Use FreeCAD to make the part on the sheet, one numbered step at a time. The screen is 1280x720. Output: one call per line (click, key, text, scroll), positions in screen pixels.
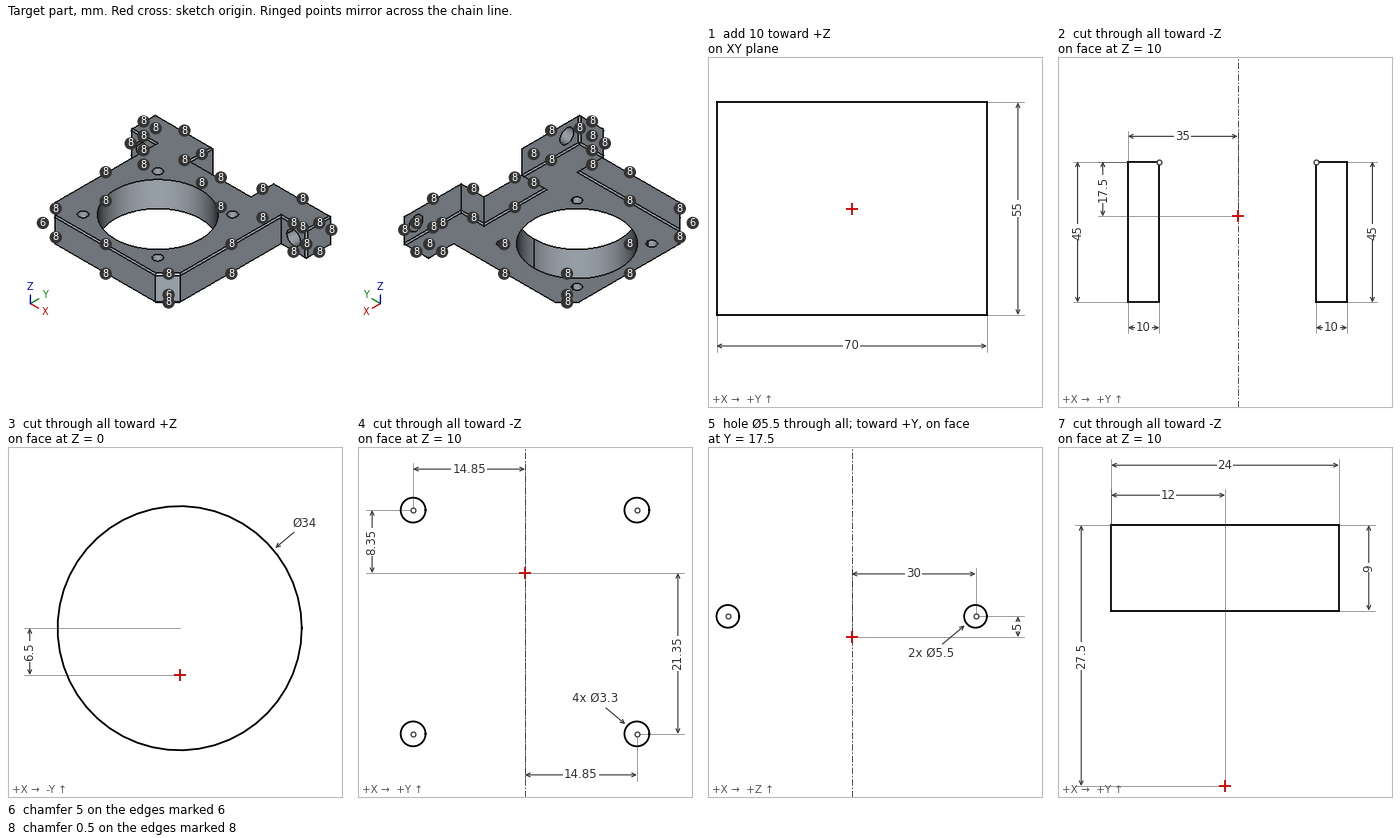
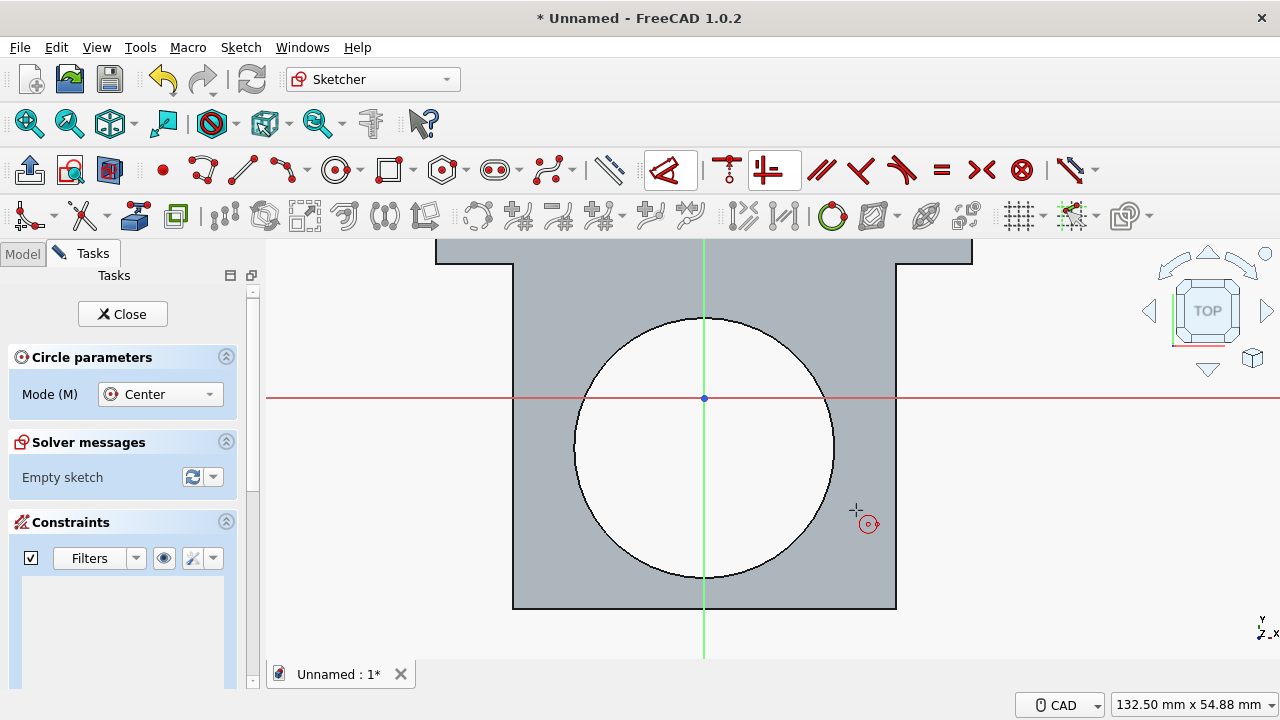
scroll(818, 562, up, 3)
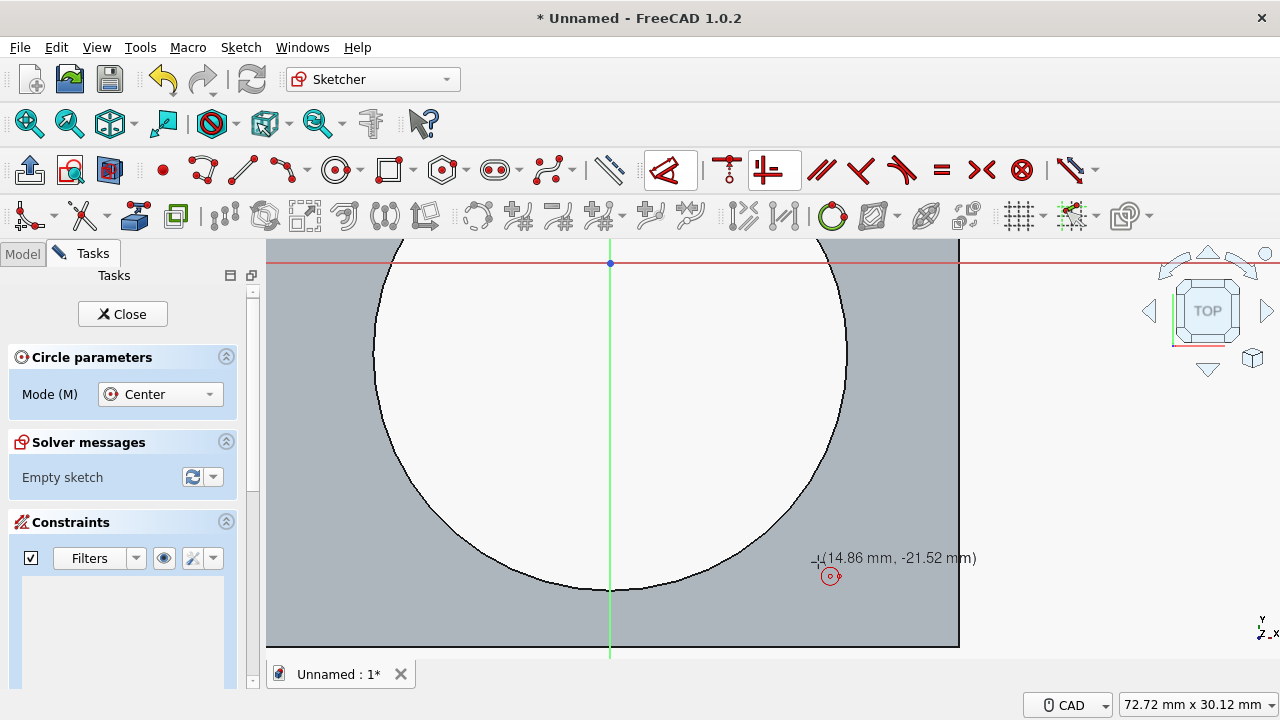
click(817, 561)
move(834, 545)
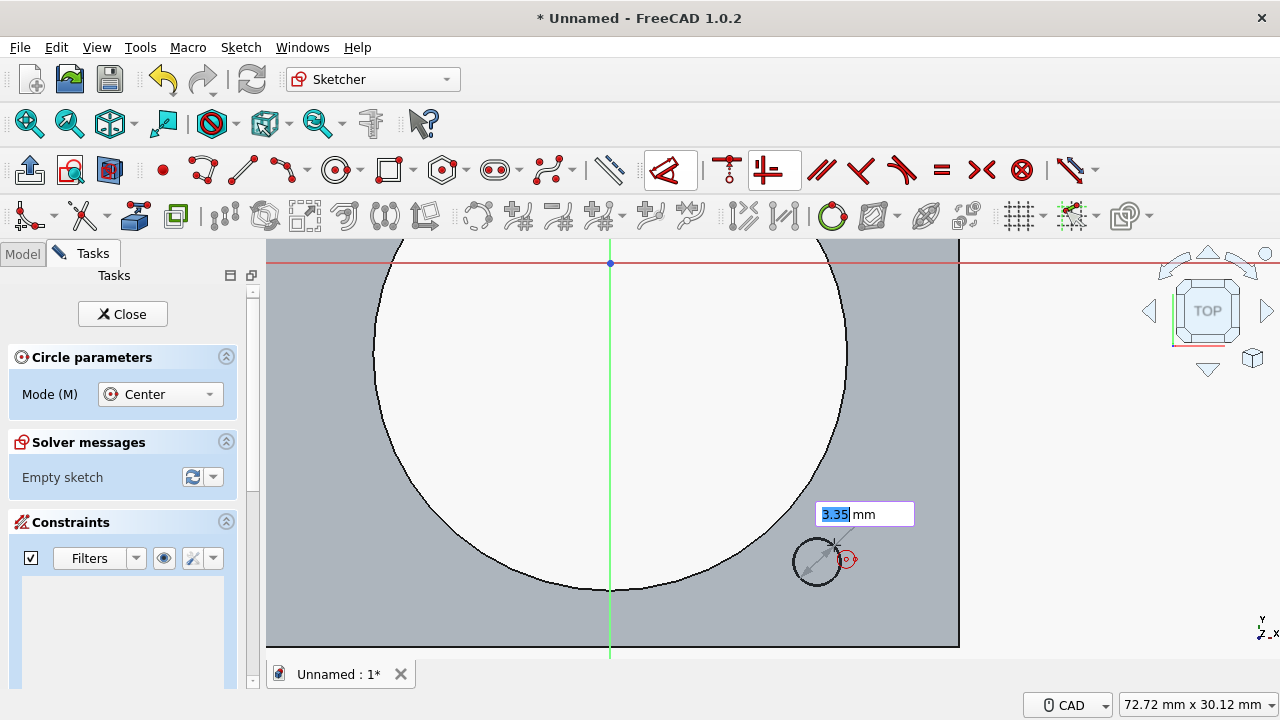
text(3.3)
key(Return)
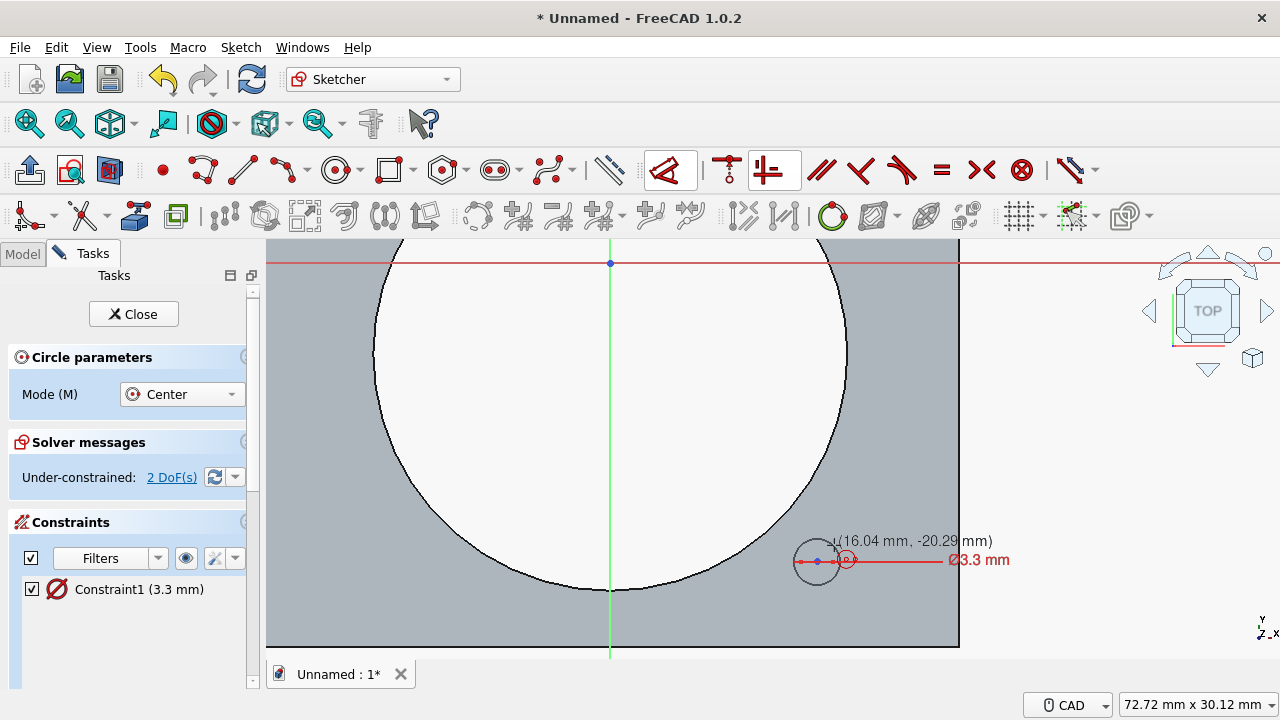
click(403, 561)
move(420, 545)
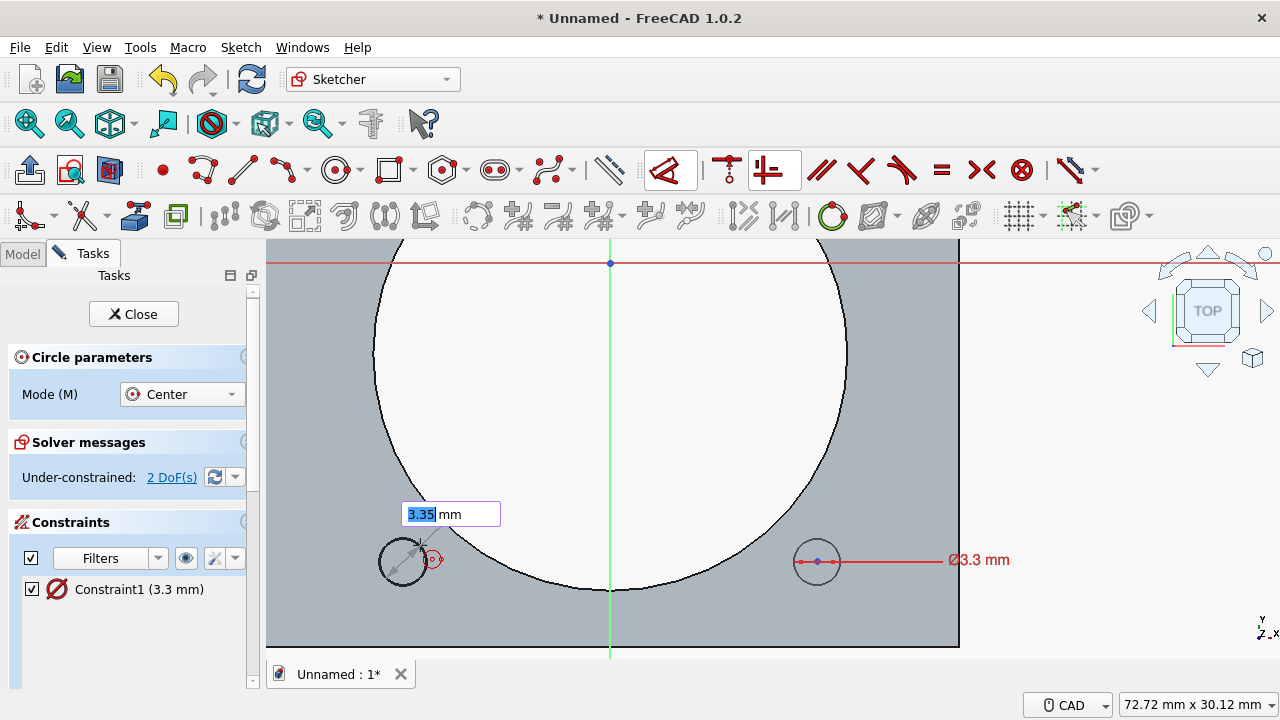
text(3.3)
key(Return)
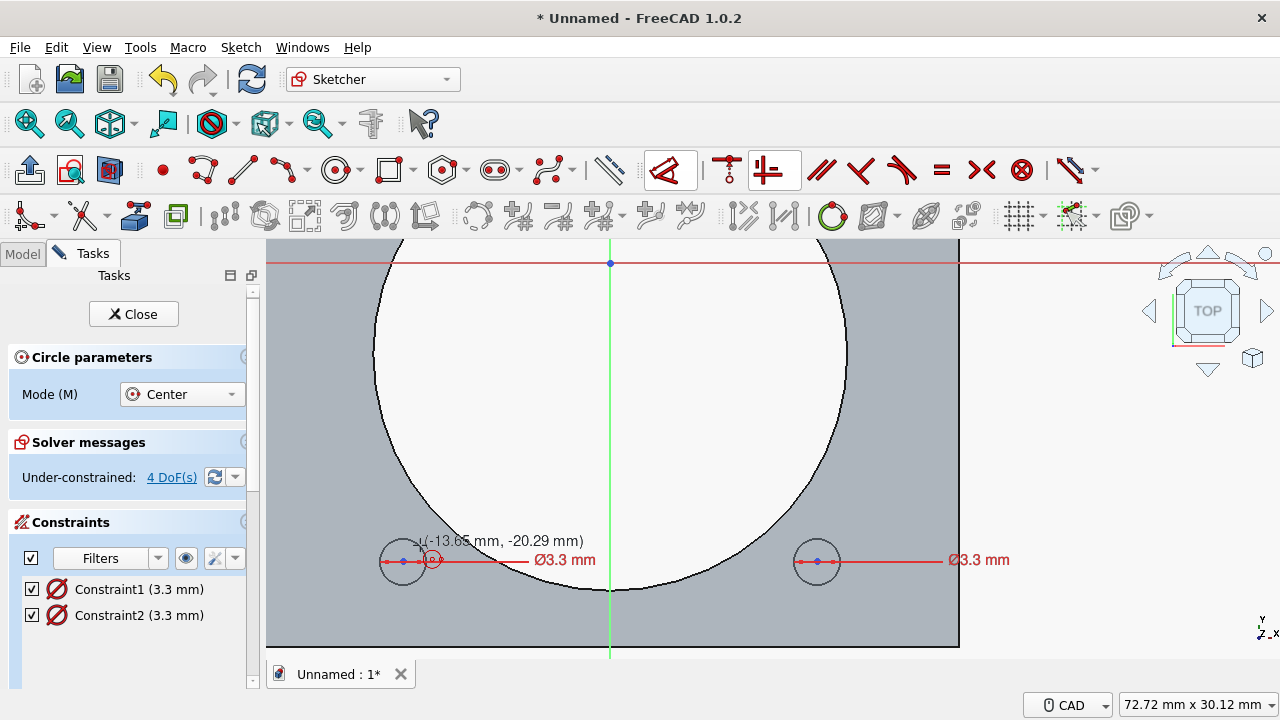
scroll(819, 565, down, 3)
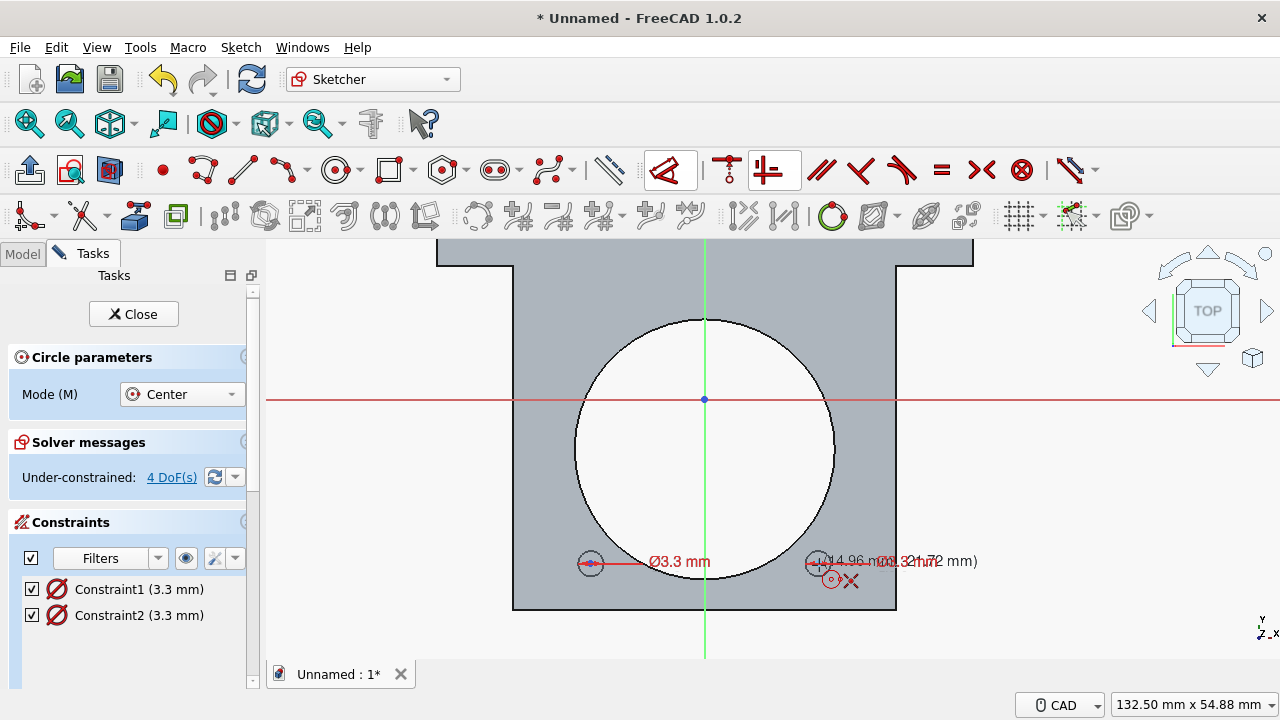
scroll(591, 336, up, 3)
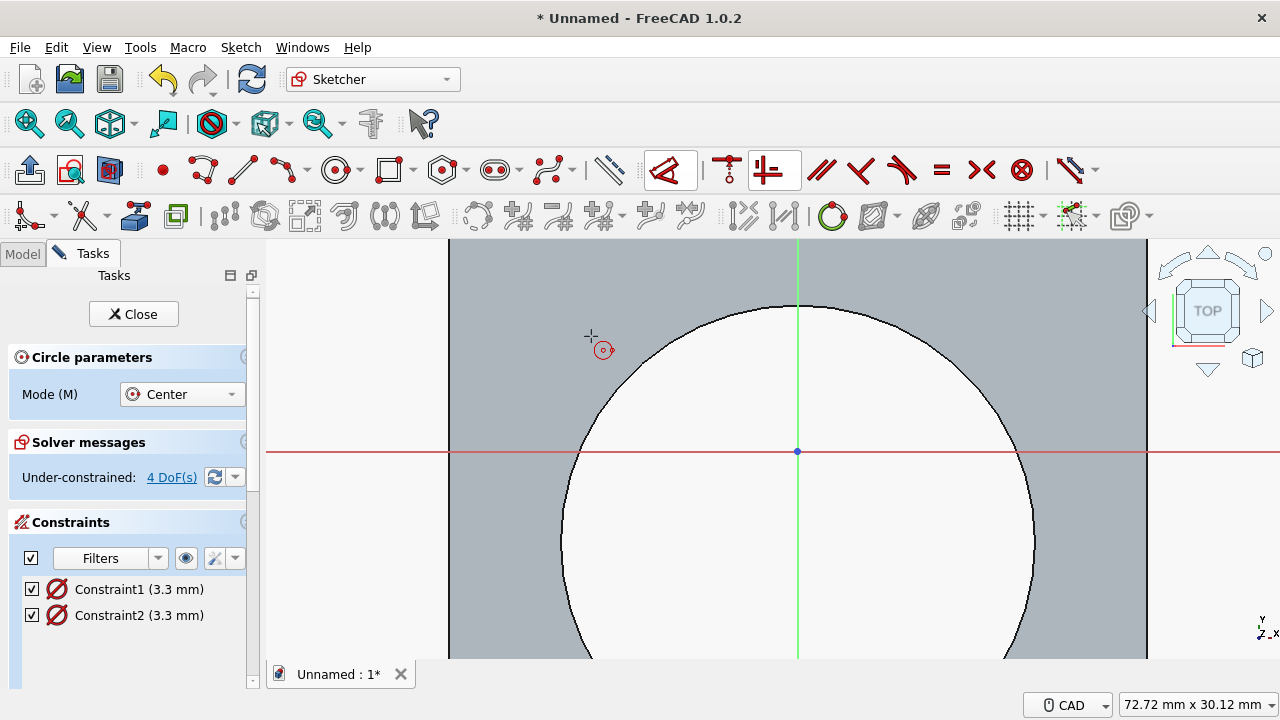
click(591, 335)
move(607, 319)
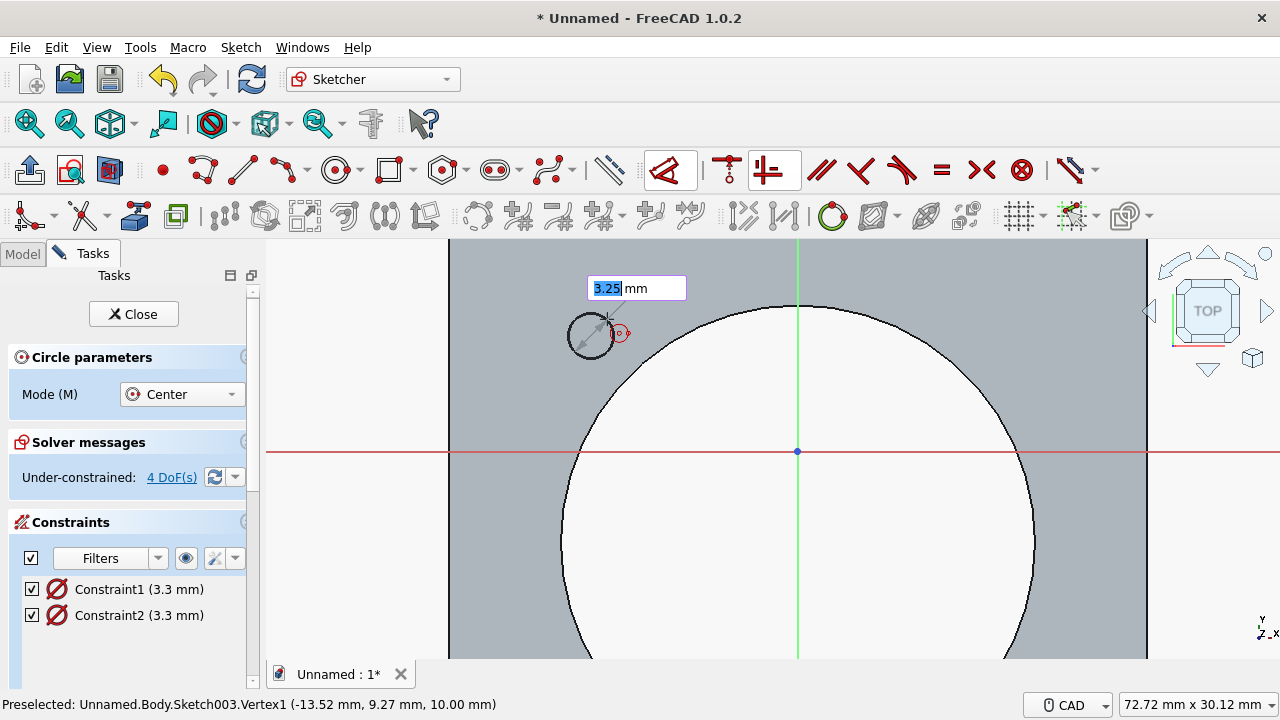
text(3.3)
key(Return)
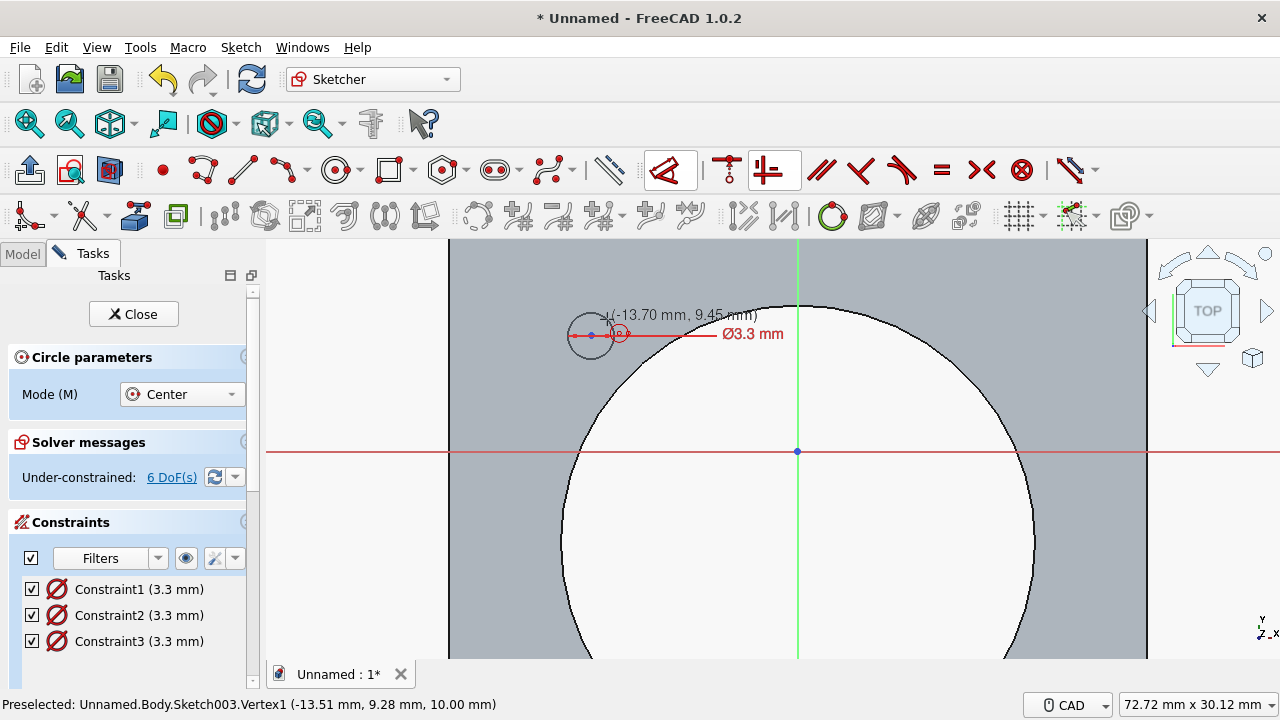
click(1005, 335)
move(1021, 319)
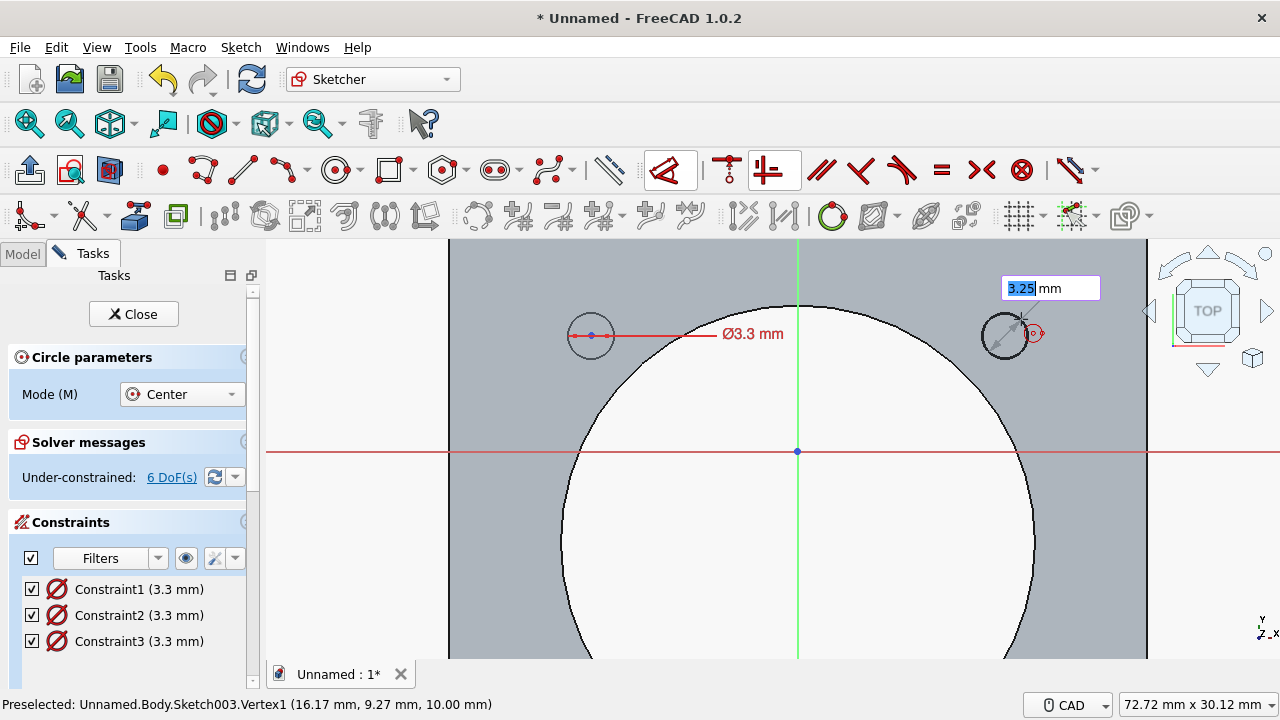
text(3.3)
key(Return)
key(Escape)